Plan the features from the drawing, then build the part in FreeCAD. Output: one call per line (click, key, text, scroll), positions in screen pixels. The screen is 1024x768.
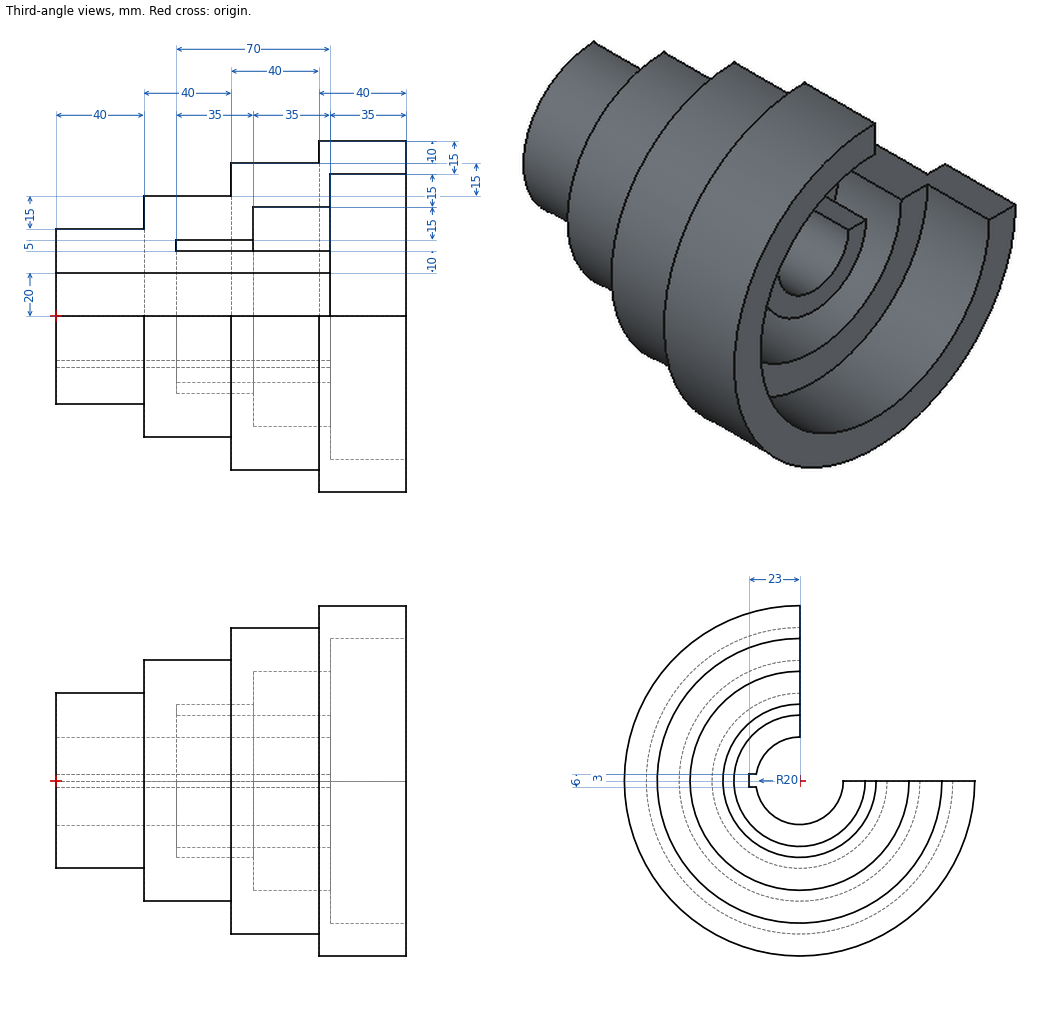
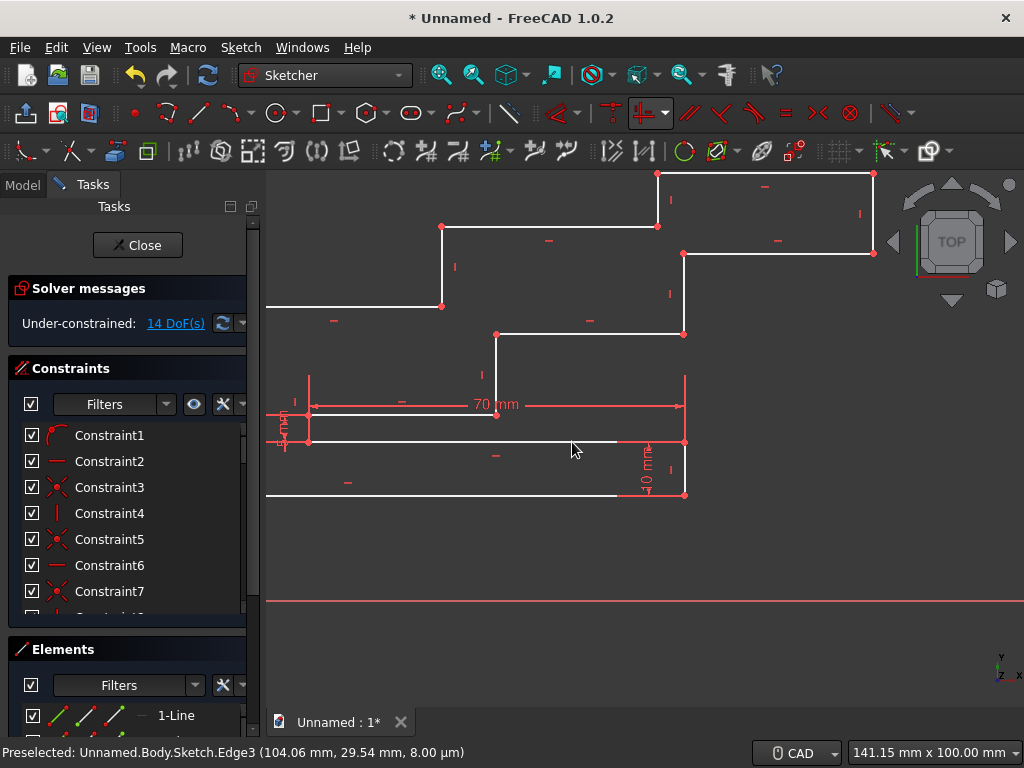
click(365, 415)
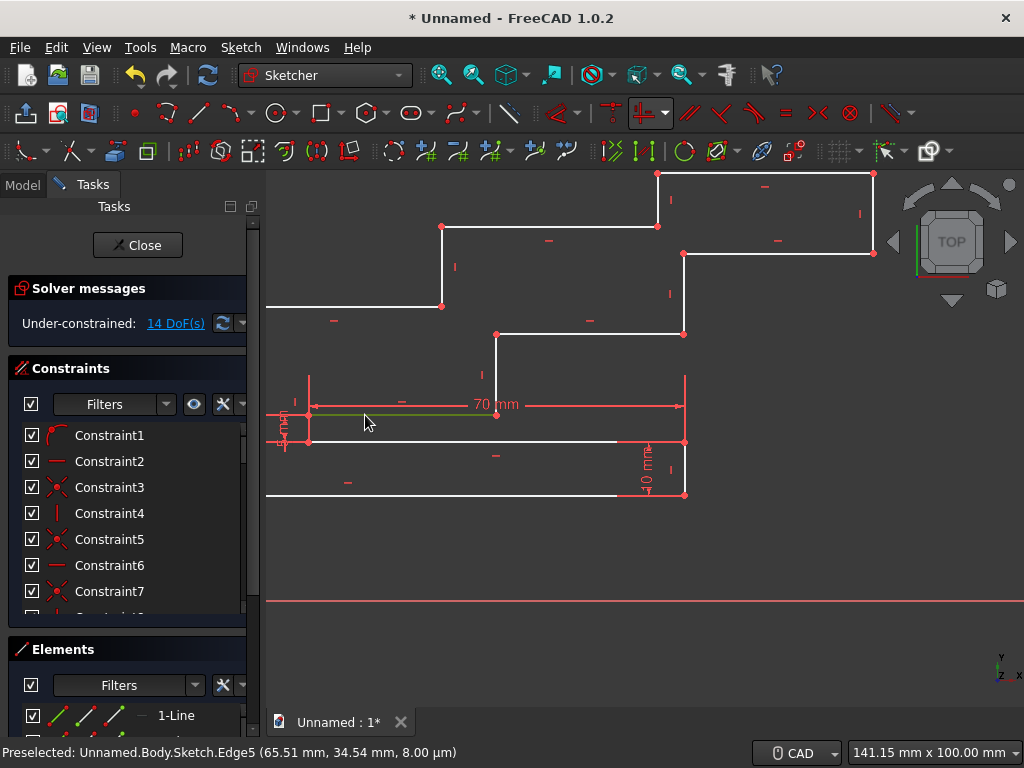
click(580, 114)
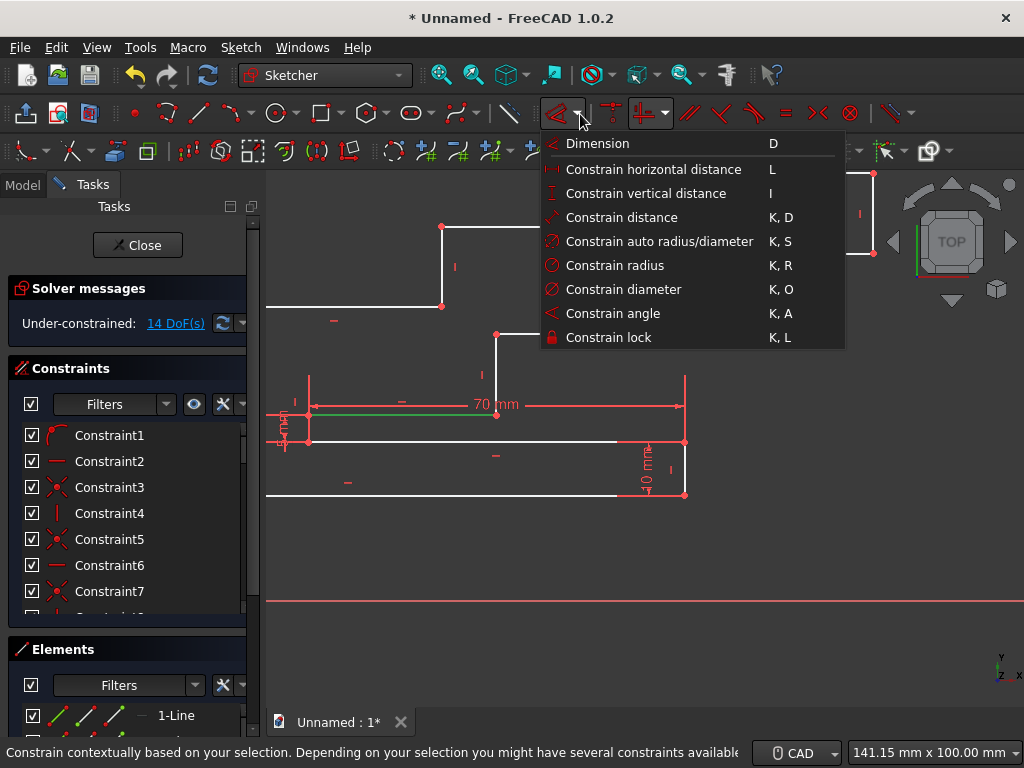
click(693, 169)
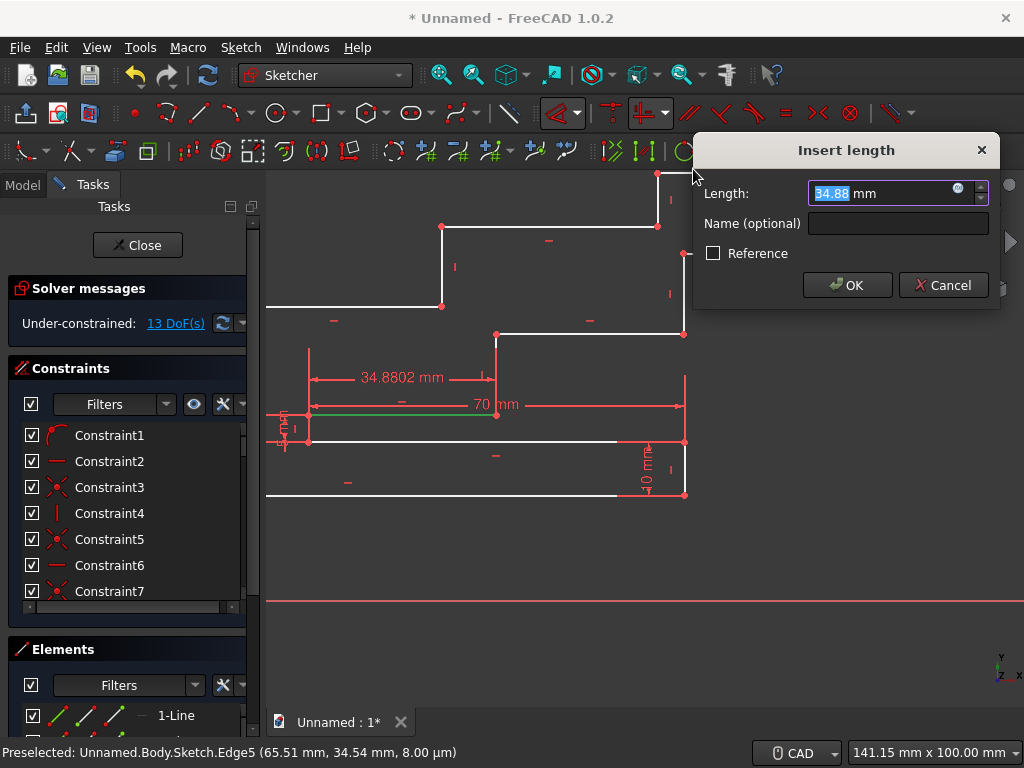
text(35)
key(Return)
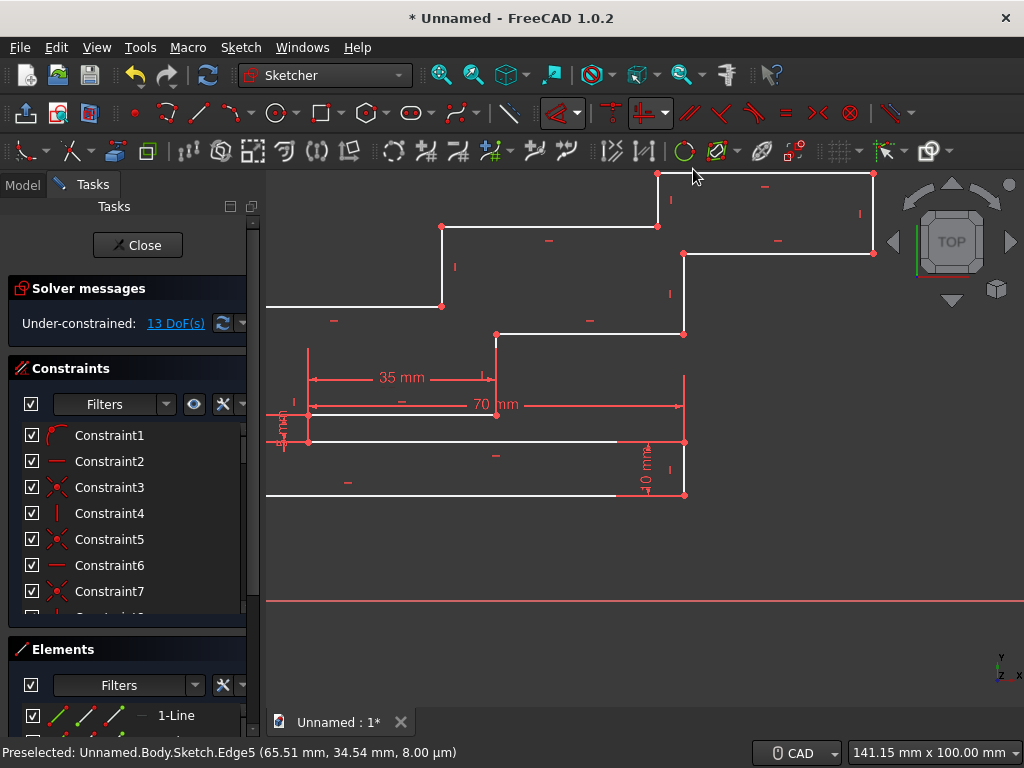
click(496, 391)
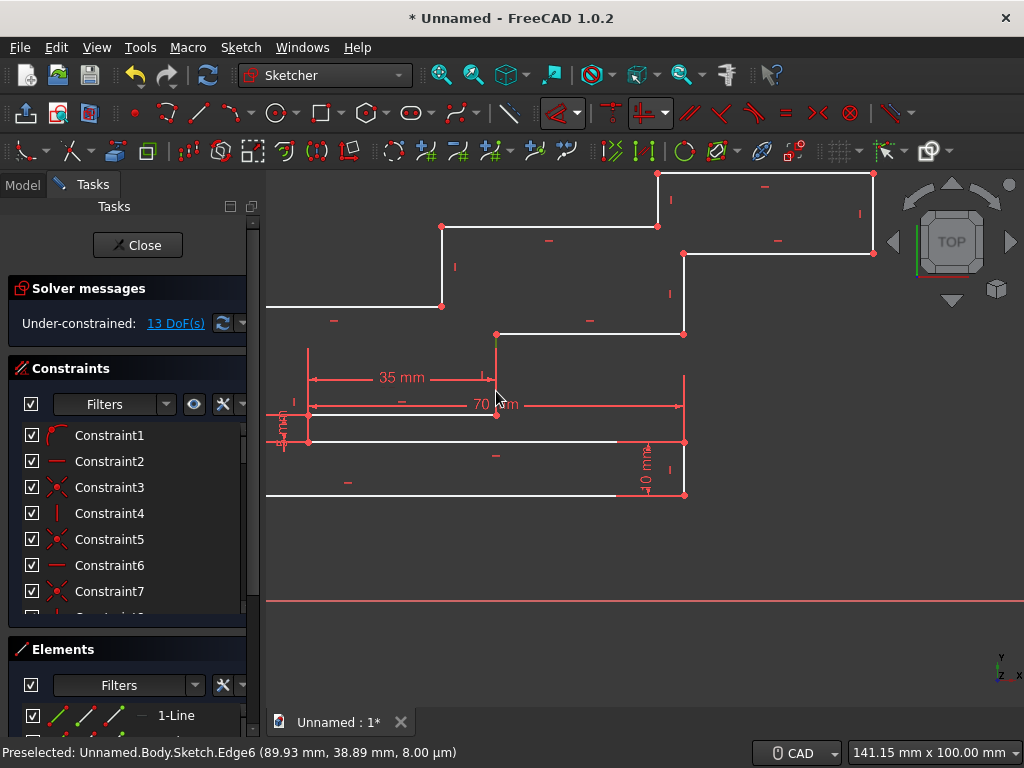
key(i)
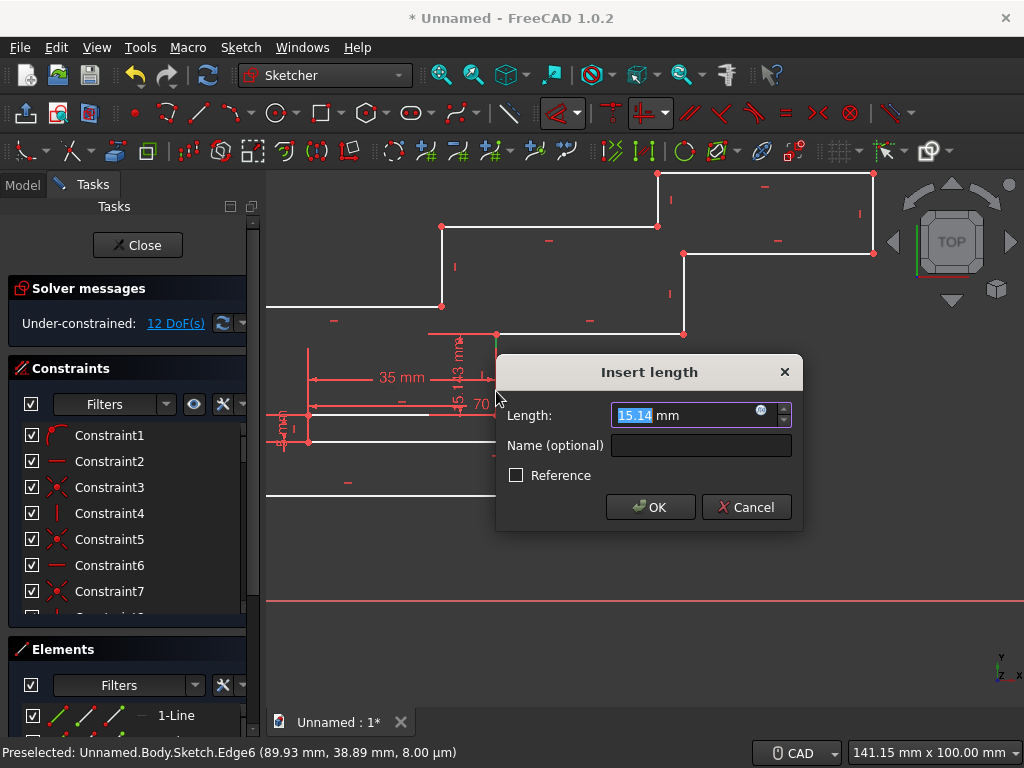
text(15)
key(Return)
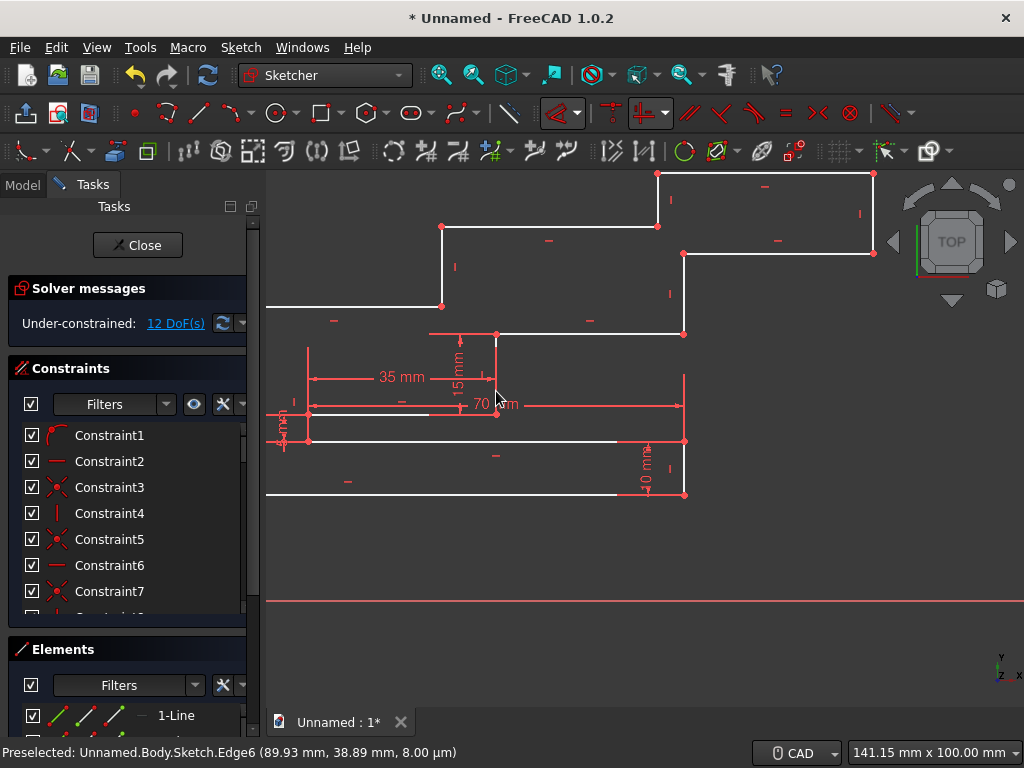
click(553, 334)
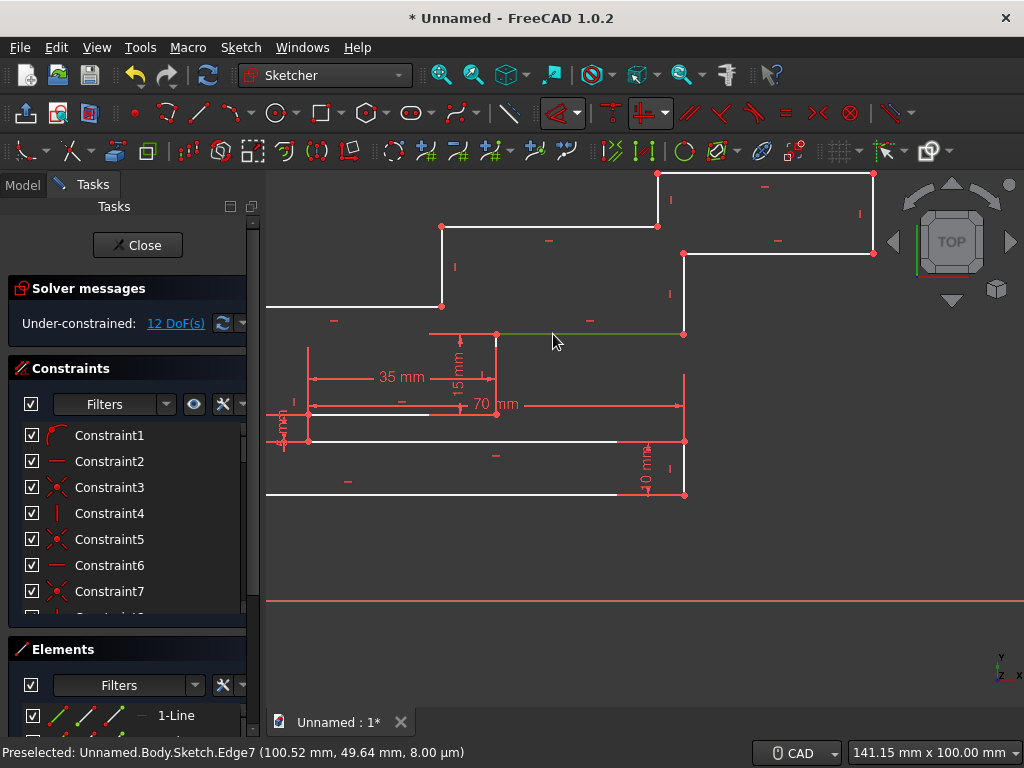
click(580, 114)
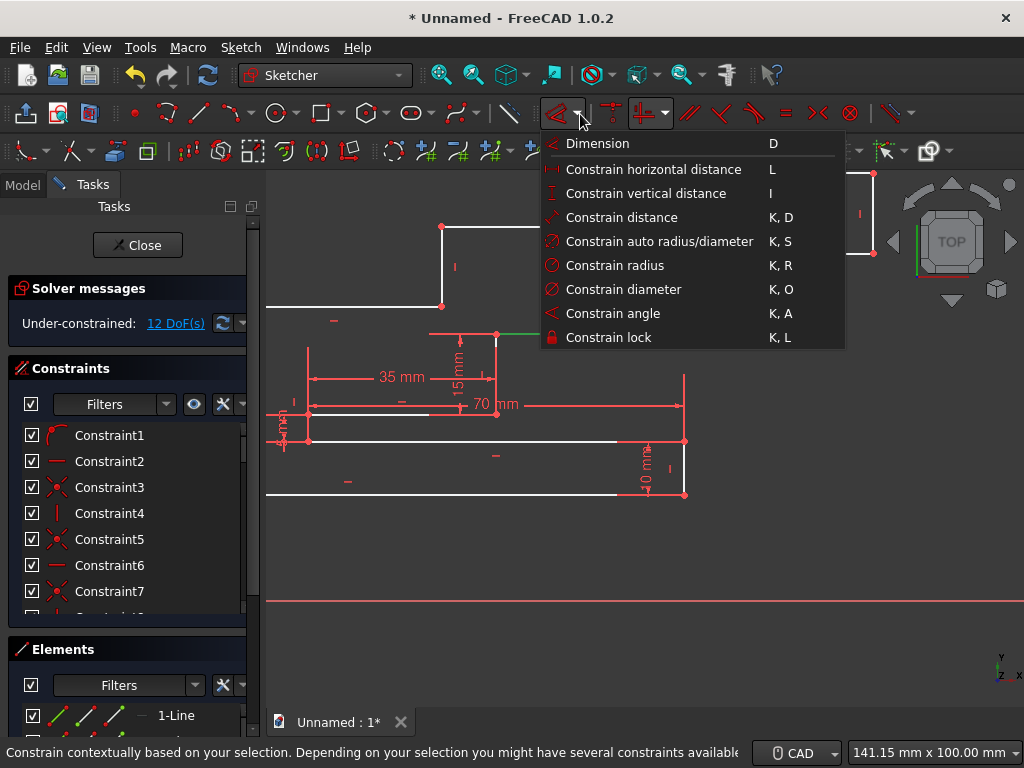
click(693, 169)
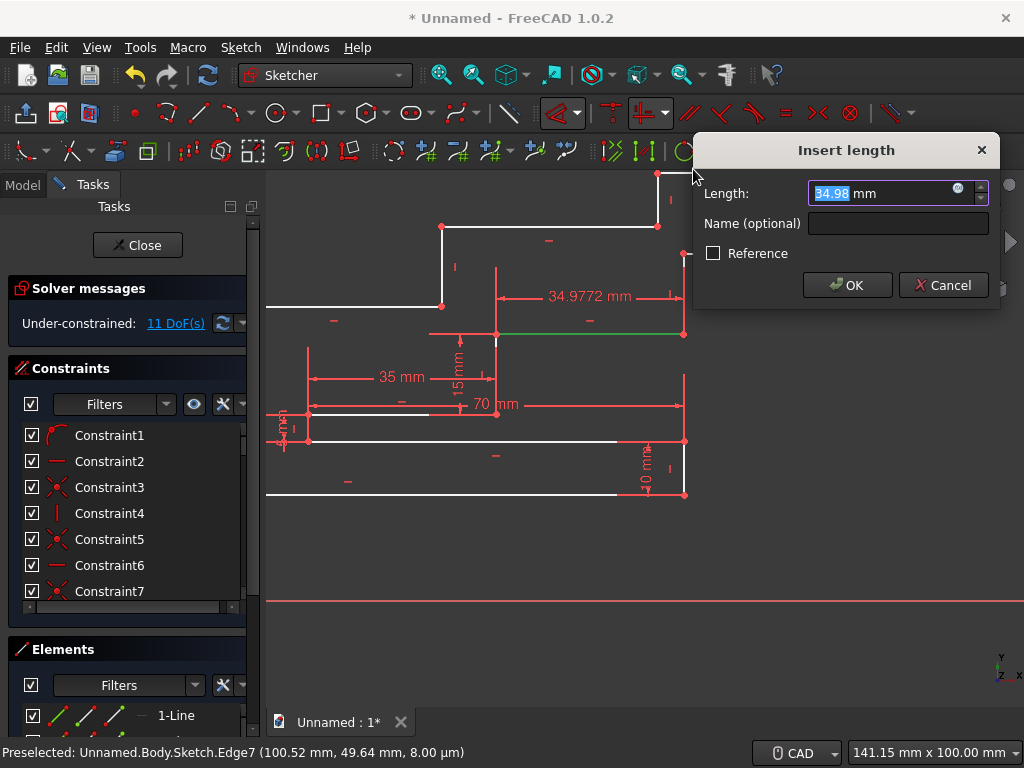
text(35)
key(Return)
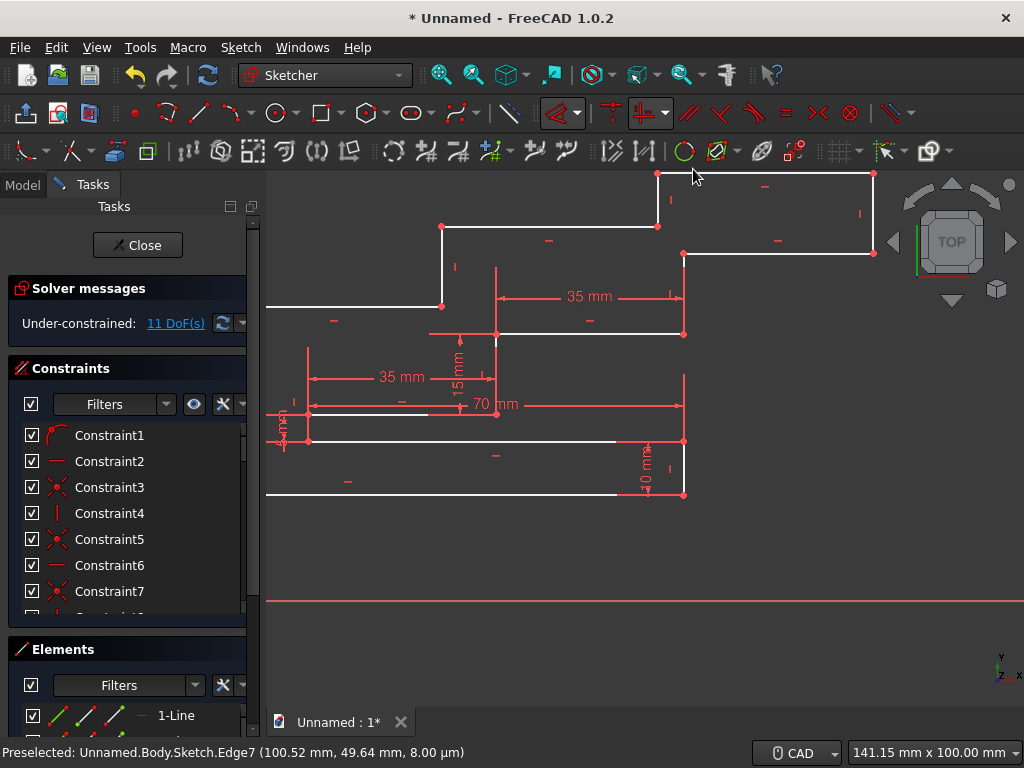
click(684, 310)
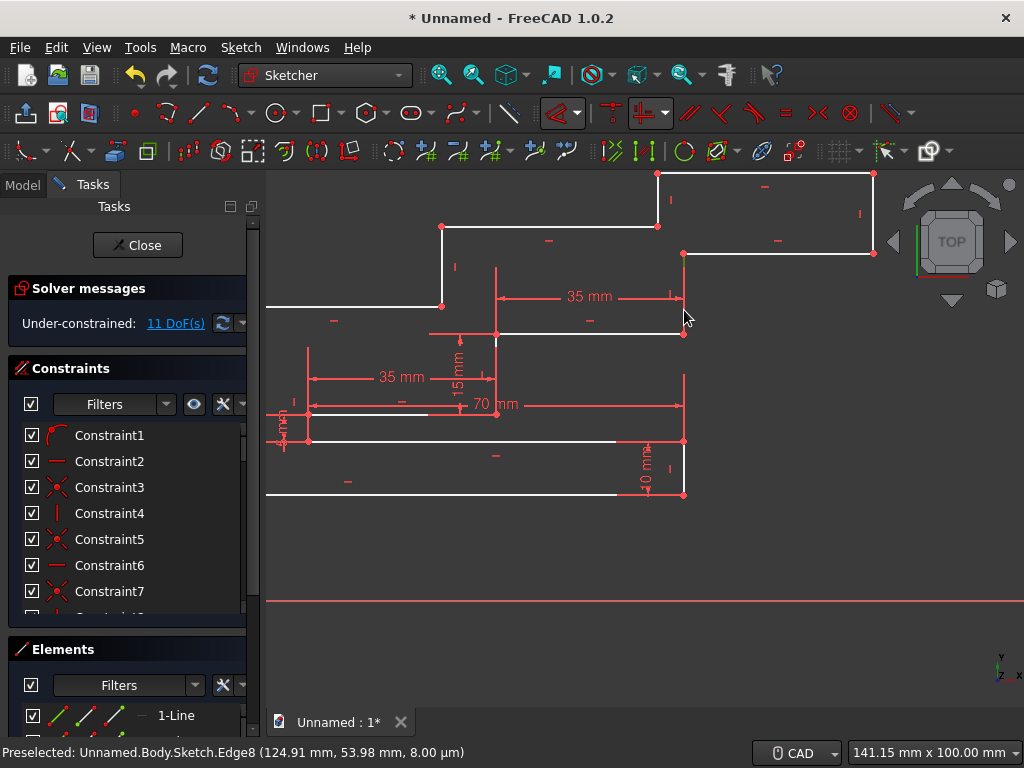
click(580, 114)